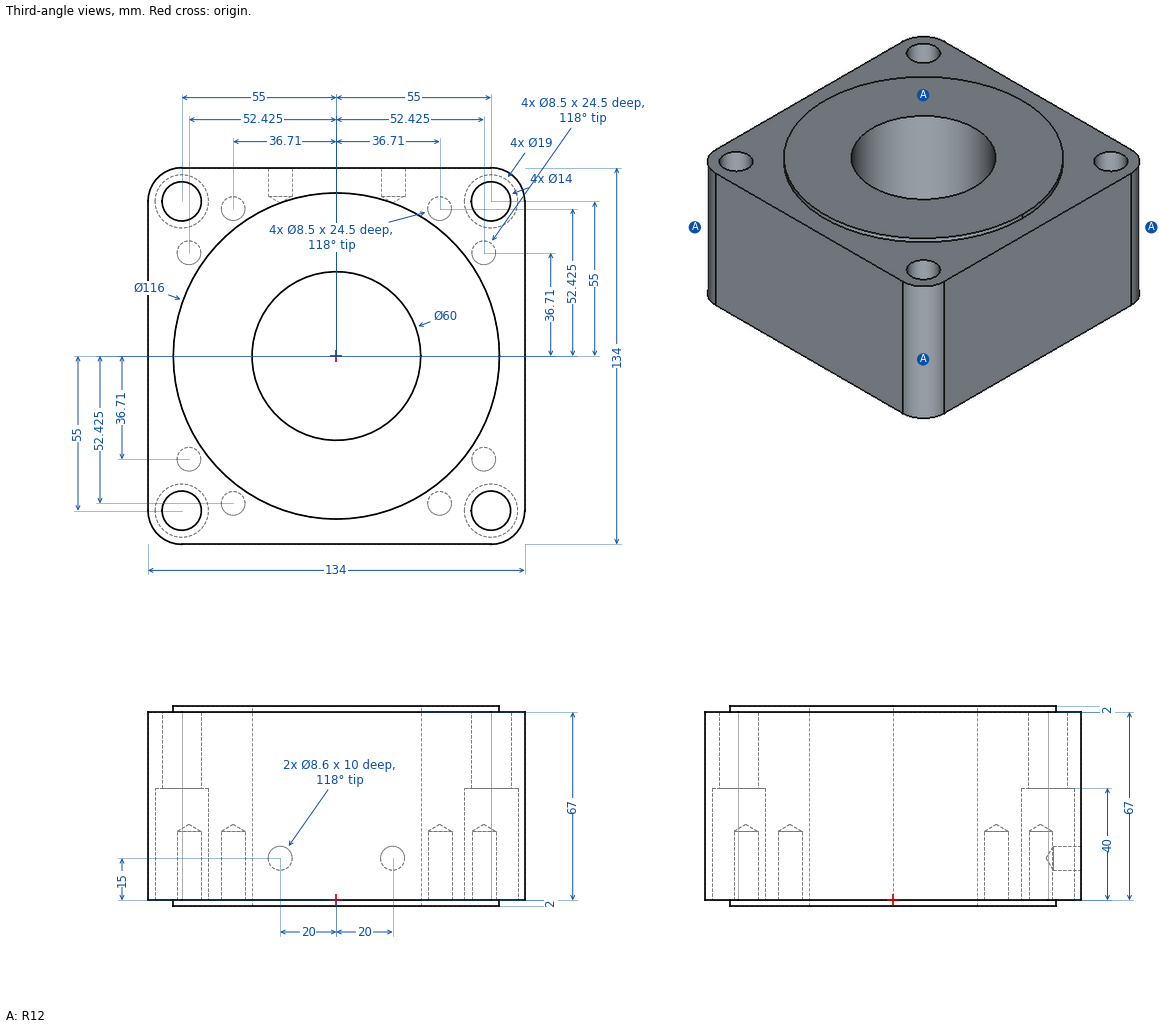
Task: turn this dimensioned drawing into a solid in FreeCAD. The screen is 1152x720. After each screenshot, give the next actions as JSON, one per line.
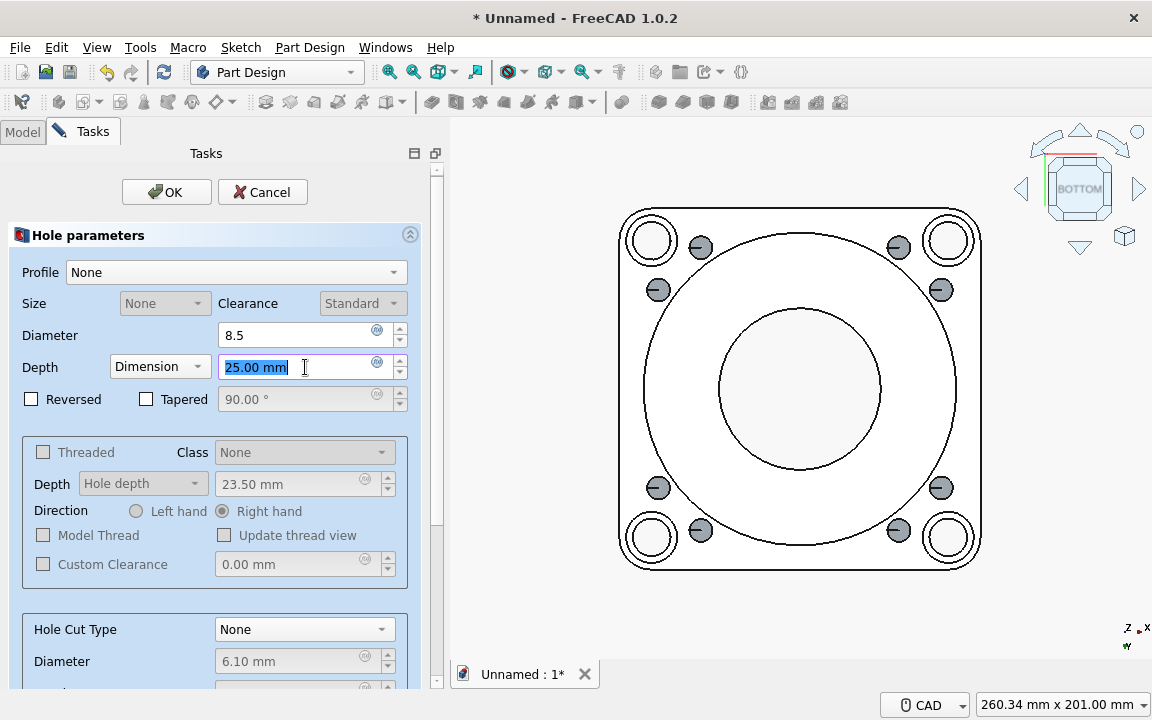
{"action": "type", "text": "24.5"}
{"action": "key", "text": "Tab"}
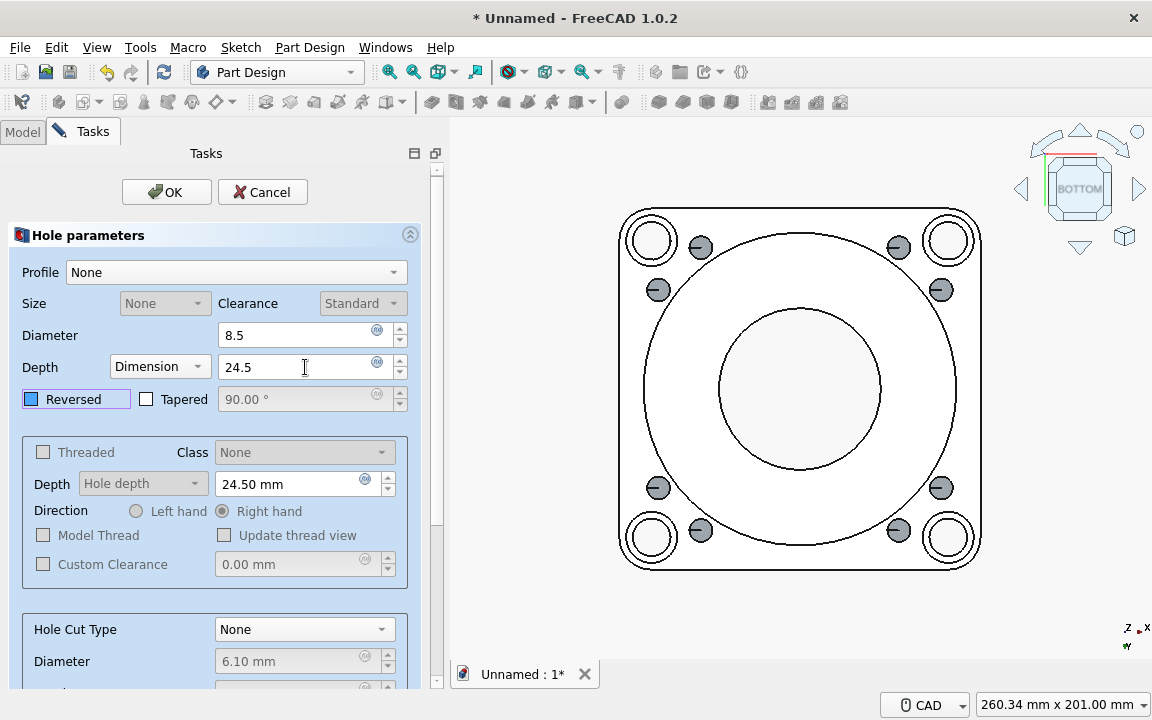
{"action": "left_click", "coordinate": [167, 192]}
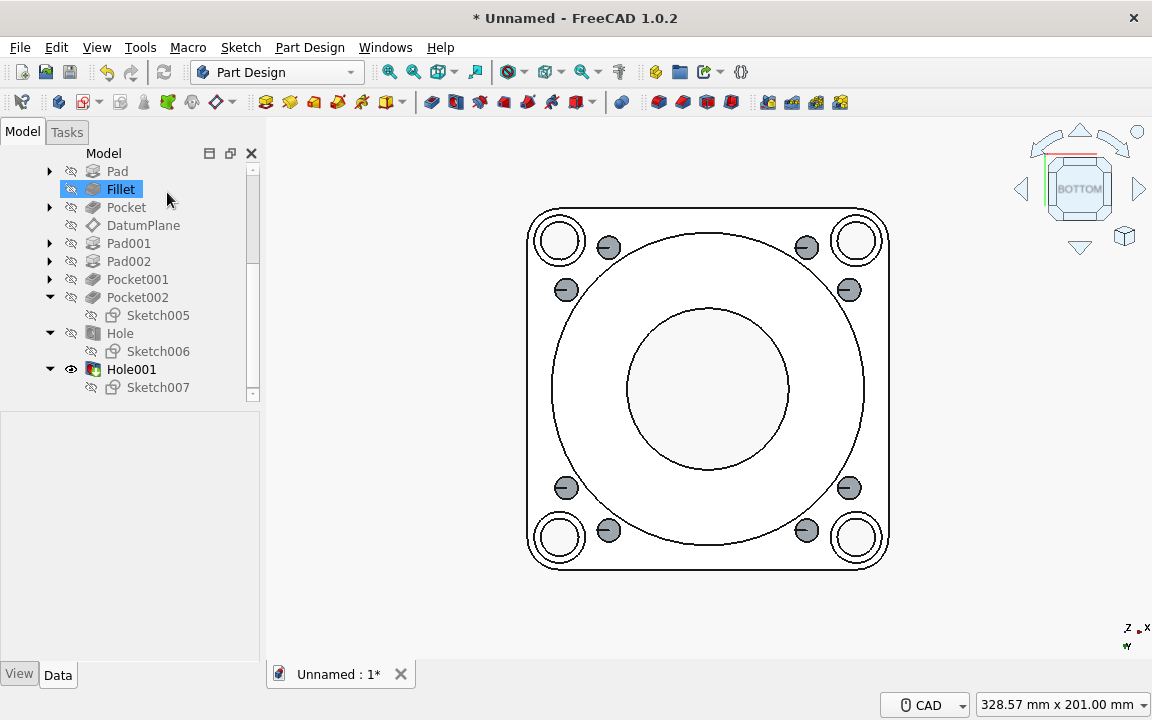
{"action": "key", "text": "4"}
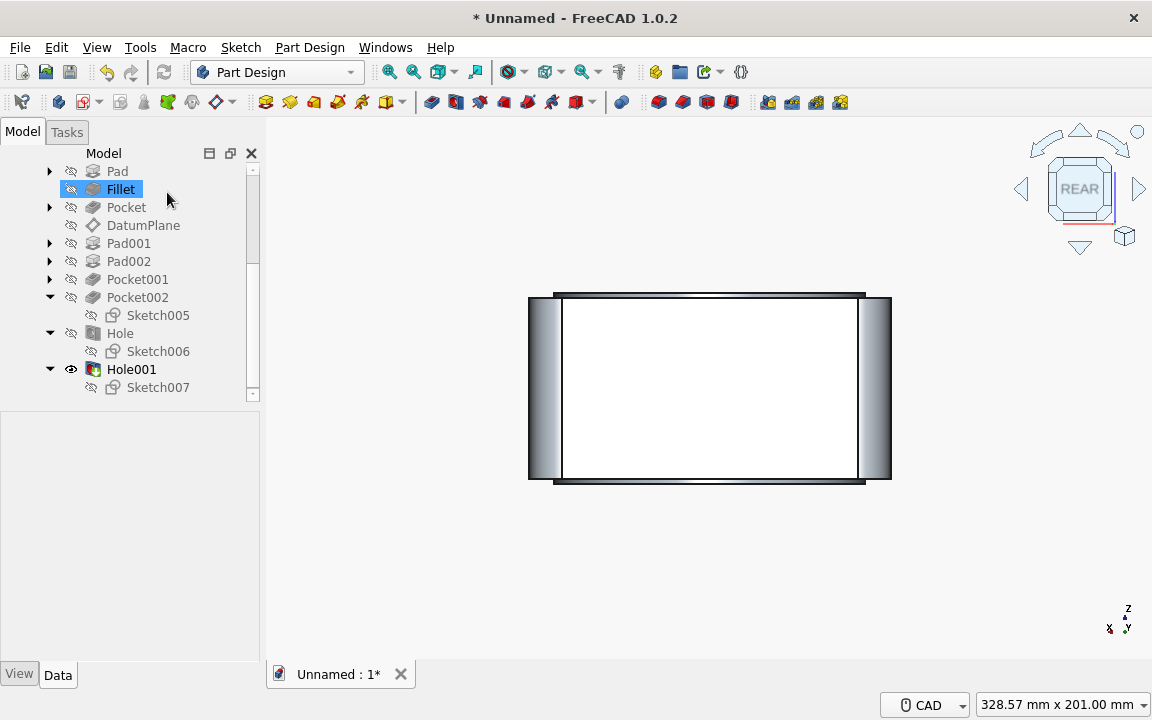
{"action": "left_click", "coordinate": [390, 72]}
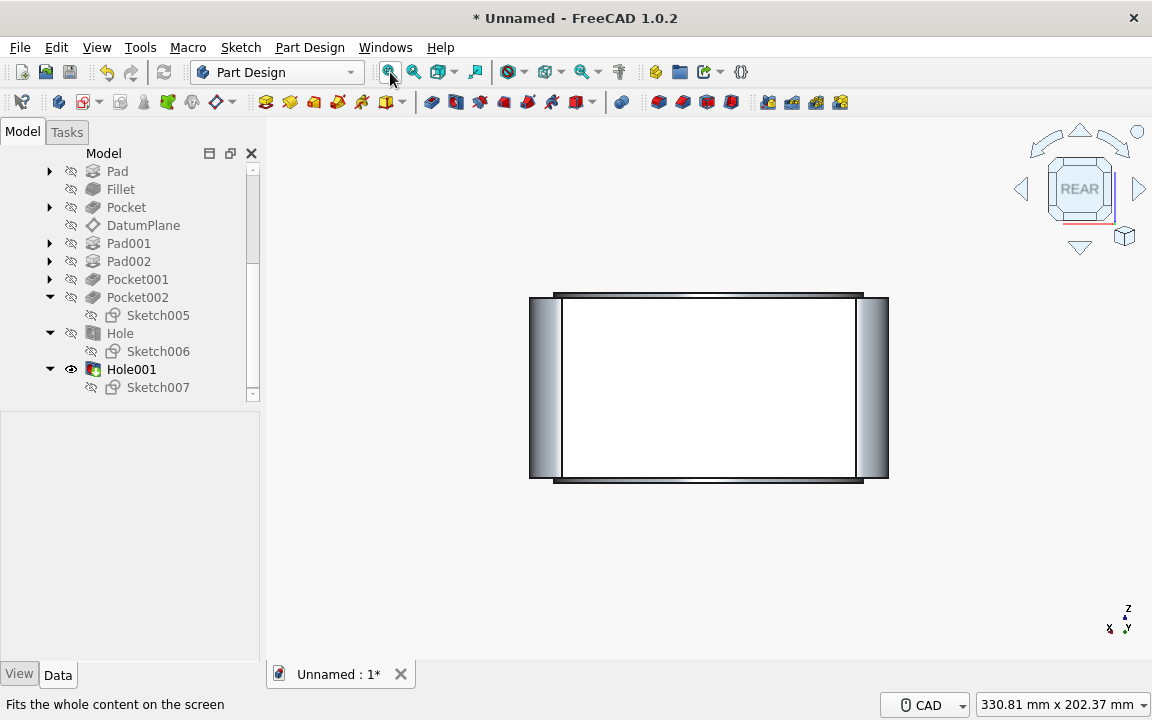
{"action": "left_click", "coordinate": [667, 387]}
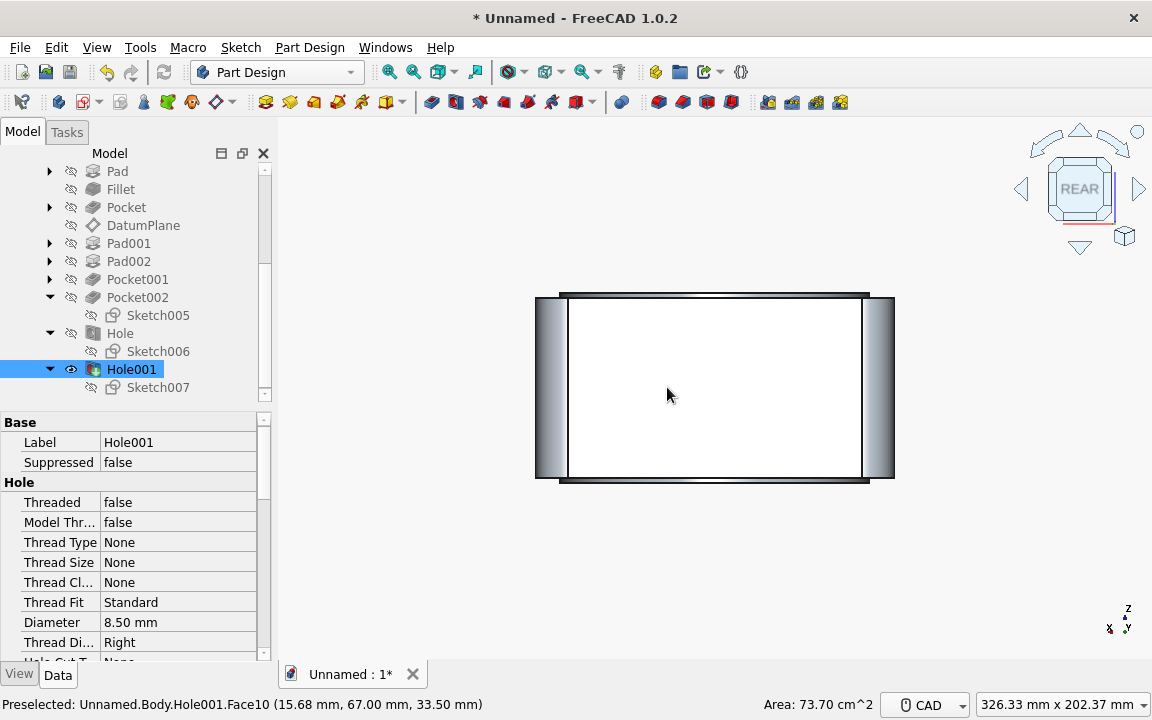
{"action": "left_click", "coordinate": [84, 102]}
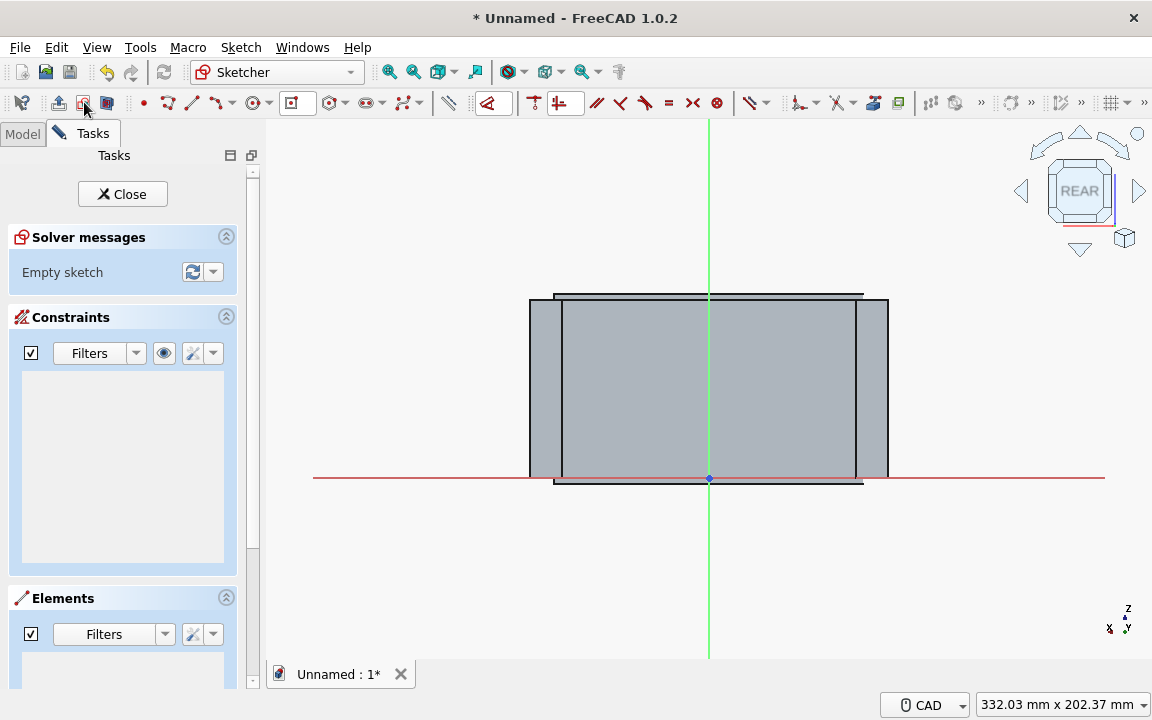
{"action": "scroll", "coordinate": [731, 473], "scroll_direction": "up", "scroll_amount": 7}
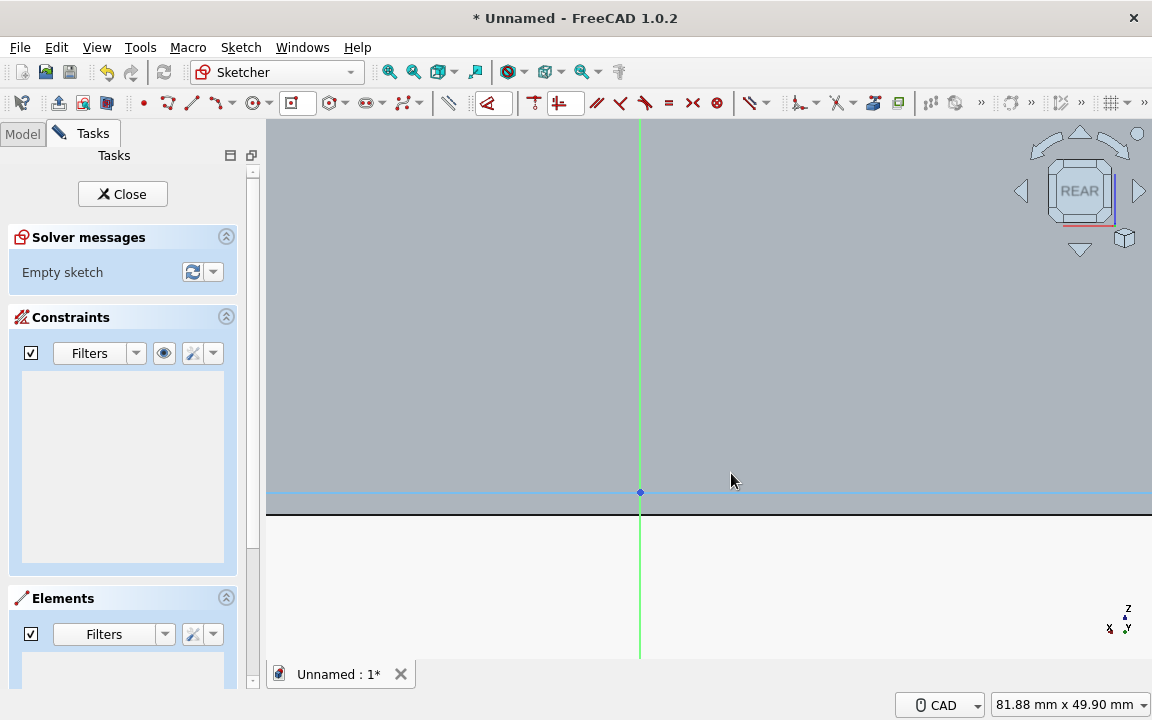
{"action": "left_click", "coordinate": [254, 104]}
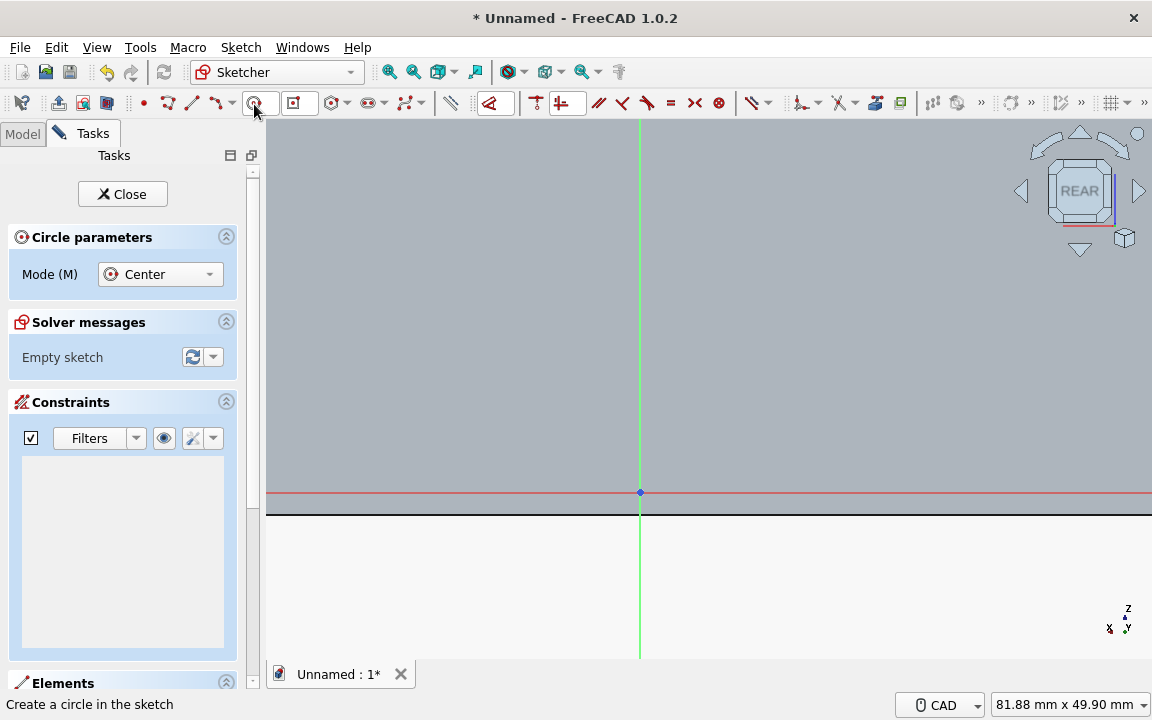
{"action": "left_click", "coordinate": [857, 331]}
{"action": "left_click", "coordinate": [889, 298]}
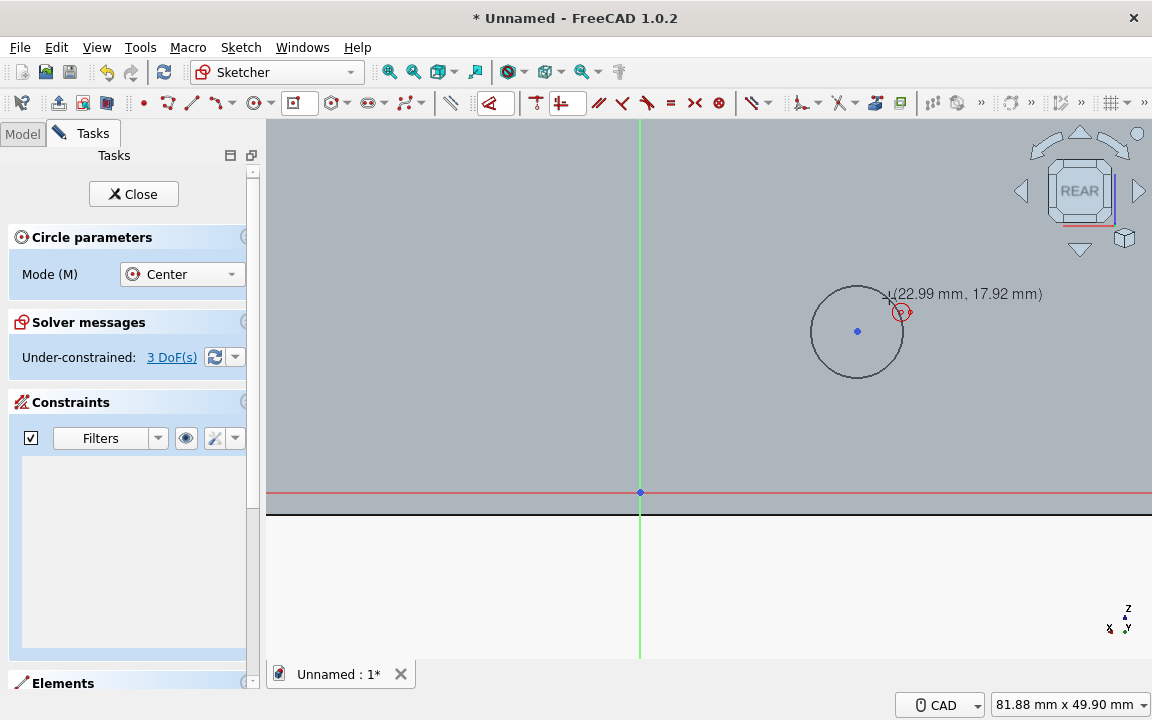
{"action": "left_click", "coordinate": [424, 331]}
{"action": "left_click", "coordinate": [457, 298]}
{"action": "key", "text": "Escape"}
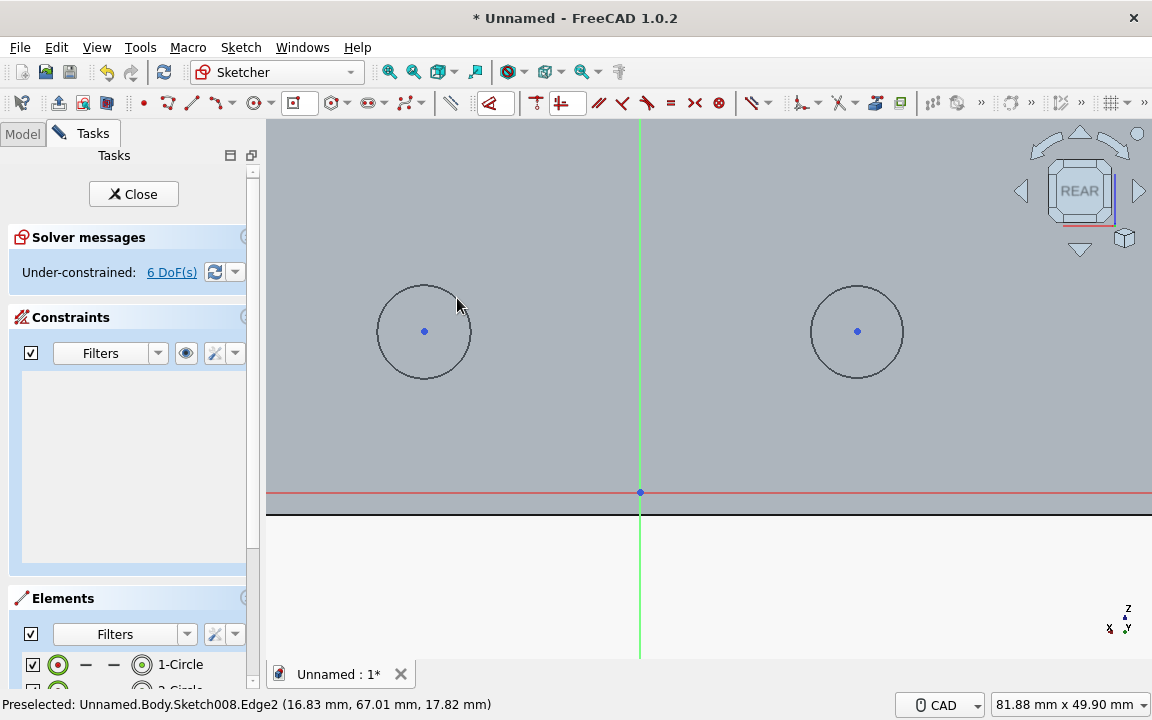
{"action": "left_click", "coordinate": [889, 299]}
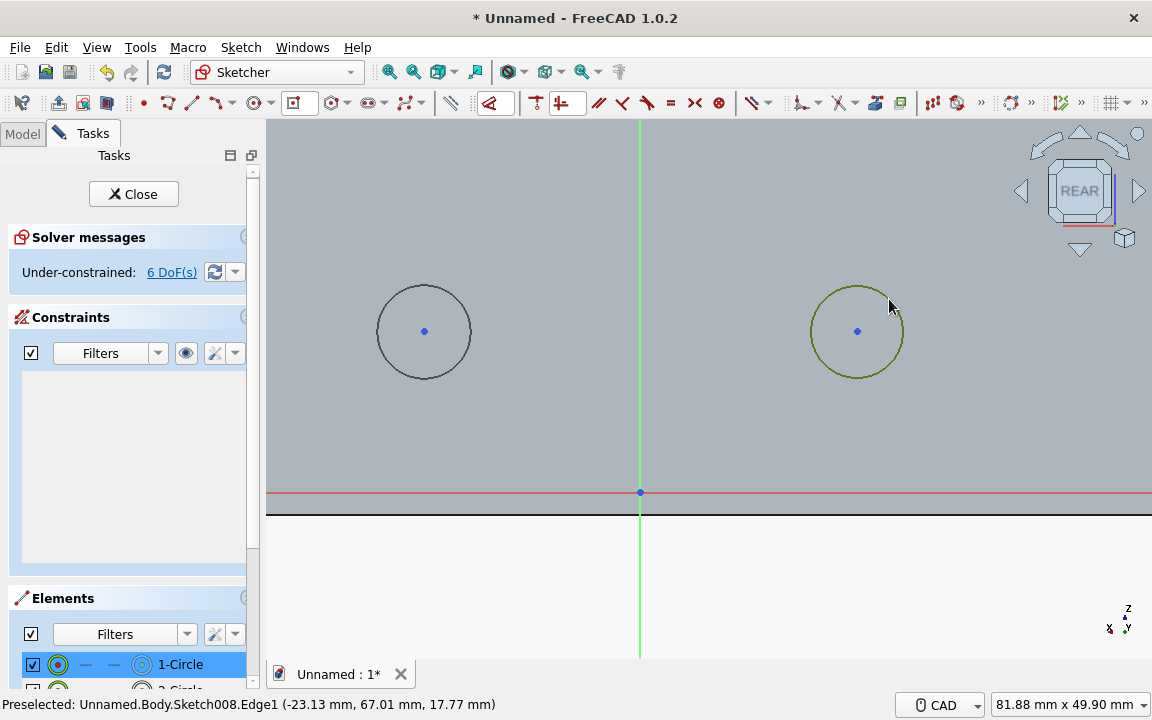
{"action": "left_click", "coordinate": [457, 299]}